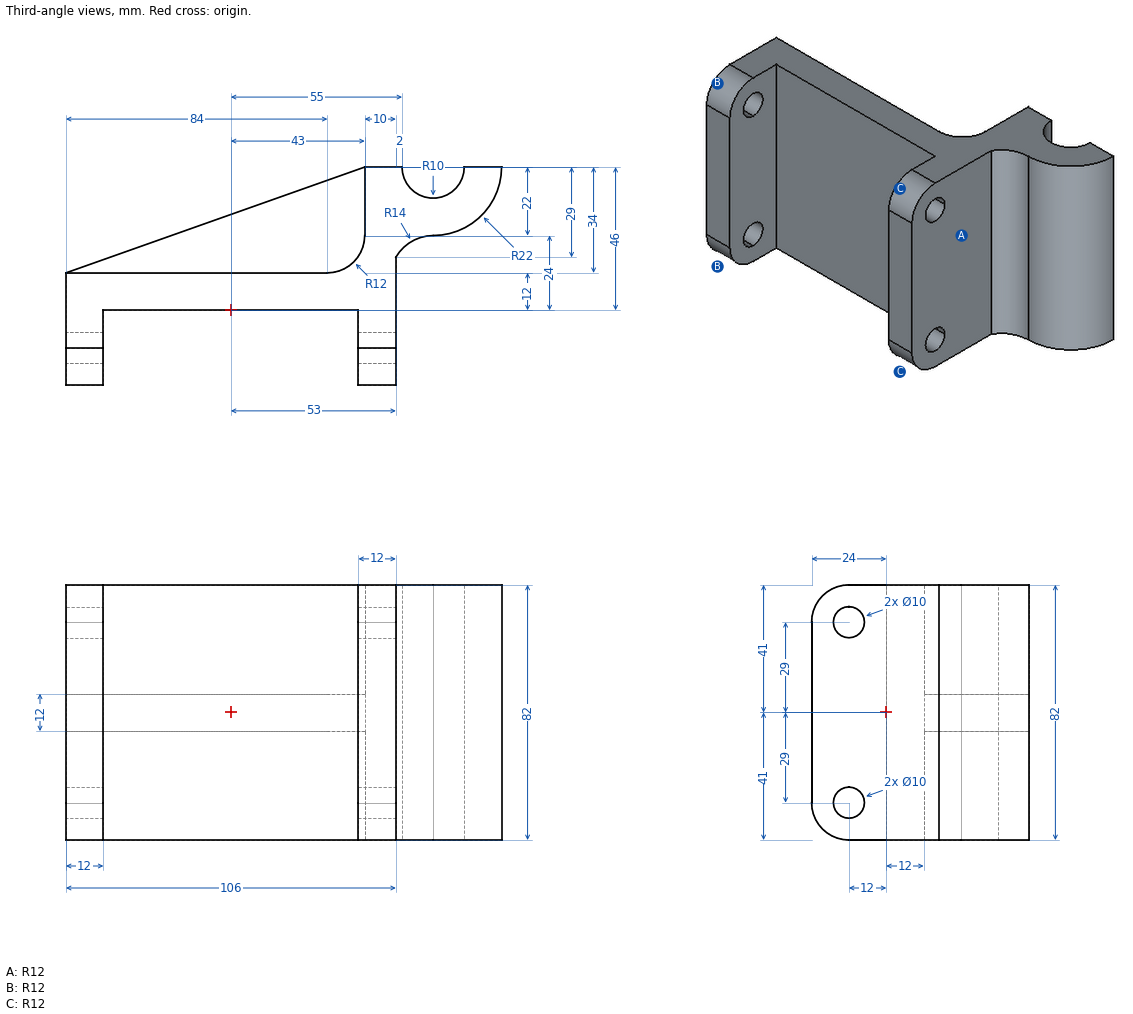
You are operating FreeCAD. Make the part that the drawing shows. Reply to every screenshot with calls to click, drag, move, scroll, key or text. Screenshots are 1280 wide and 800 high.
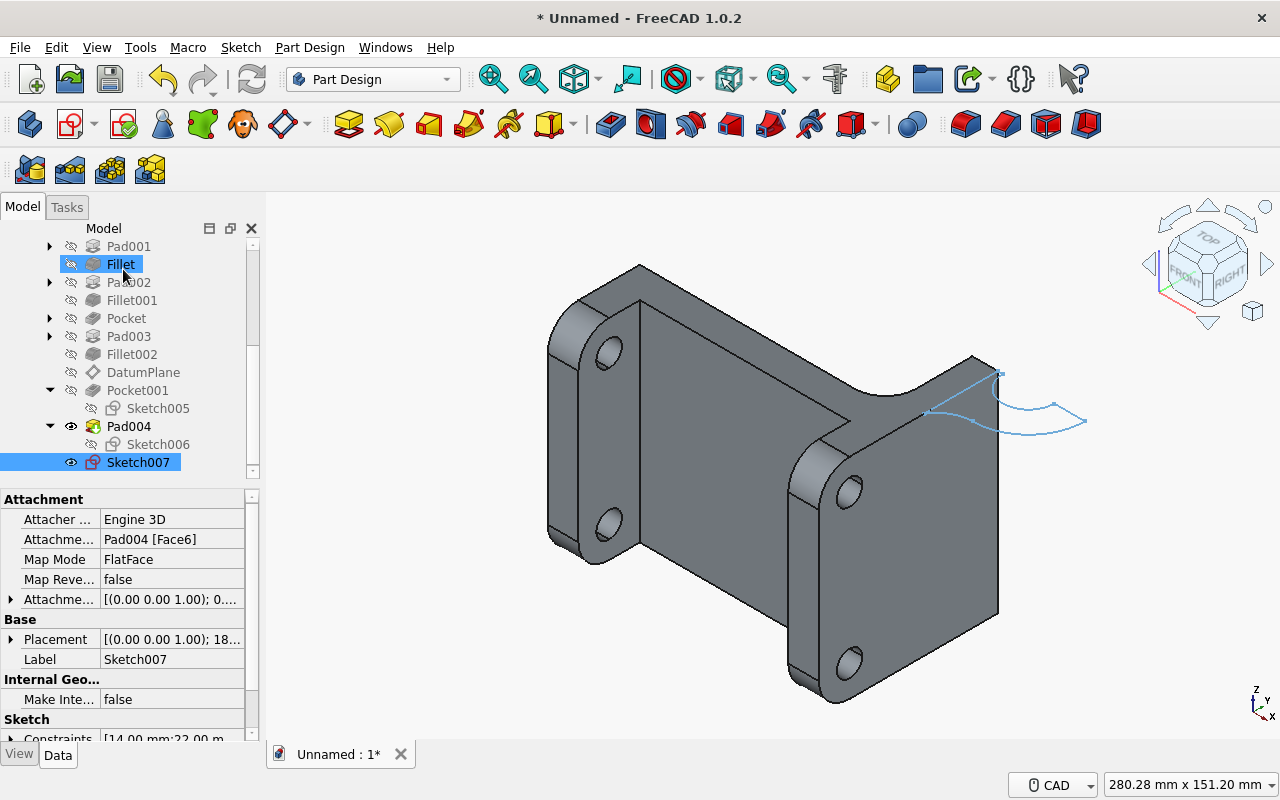
click(350, 124)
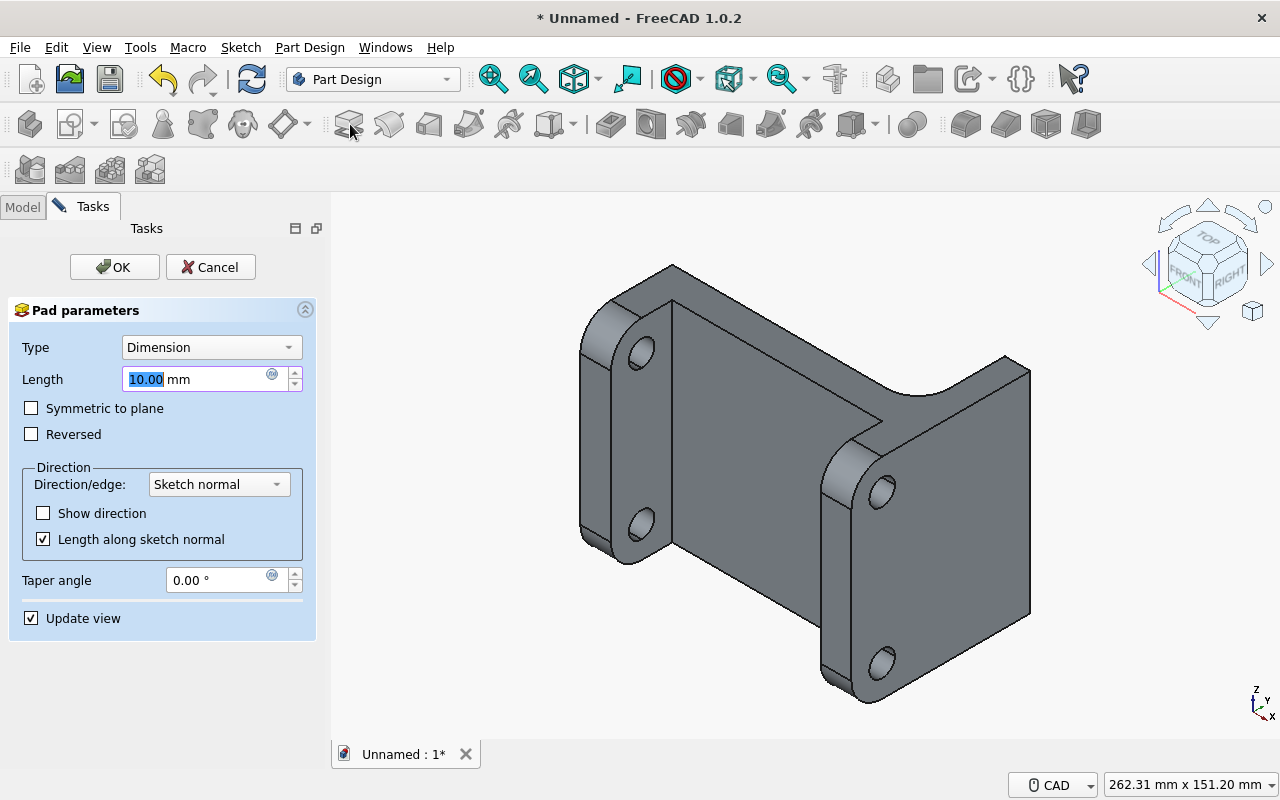
text(82)
key(Tab)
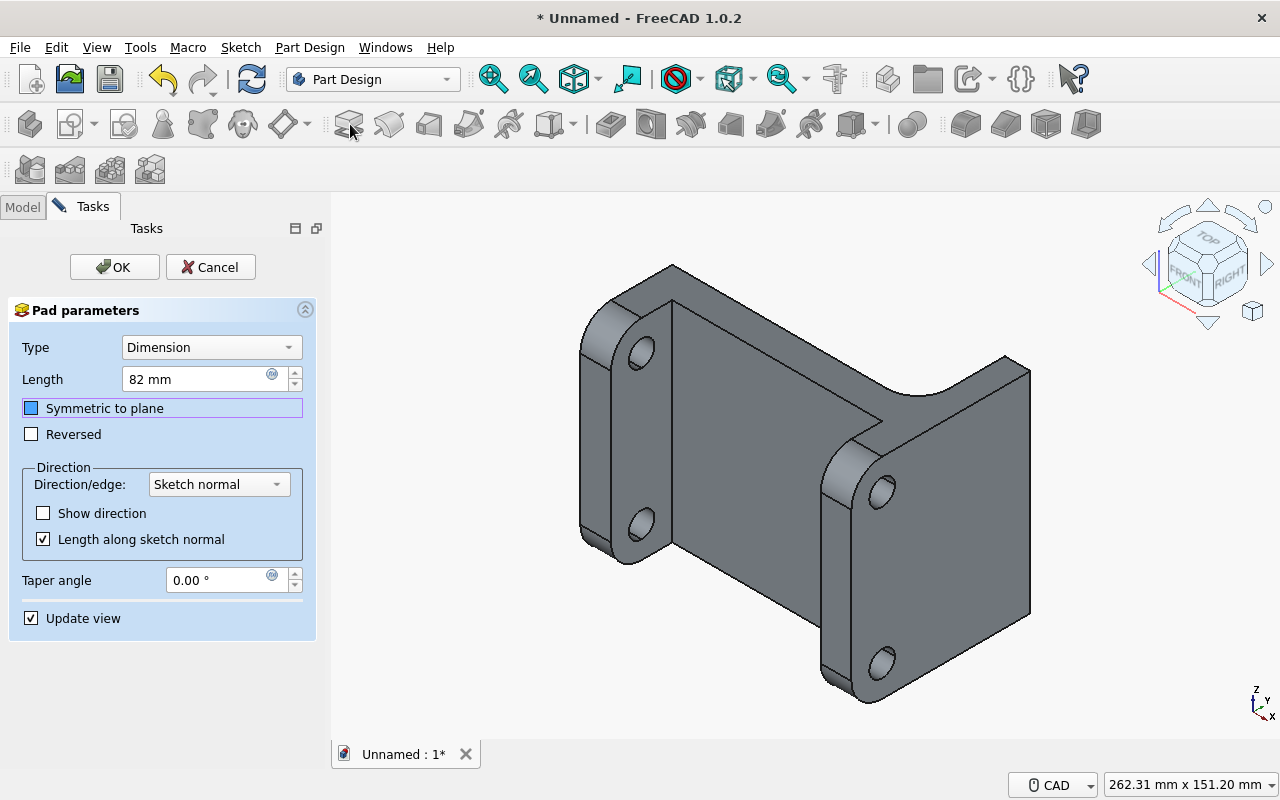
click(30, 434)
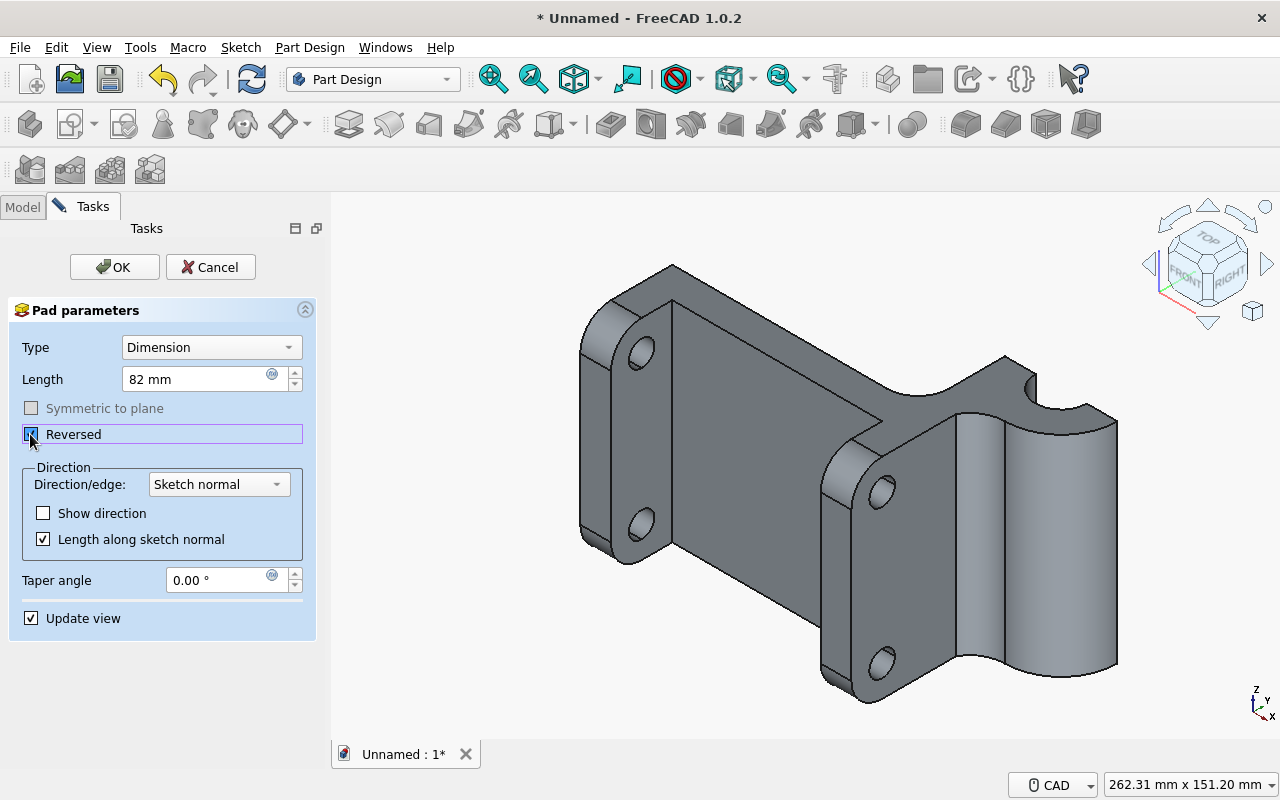
click(115, 267)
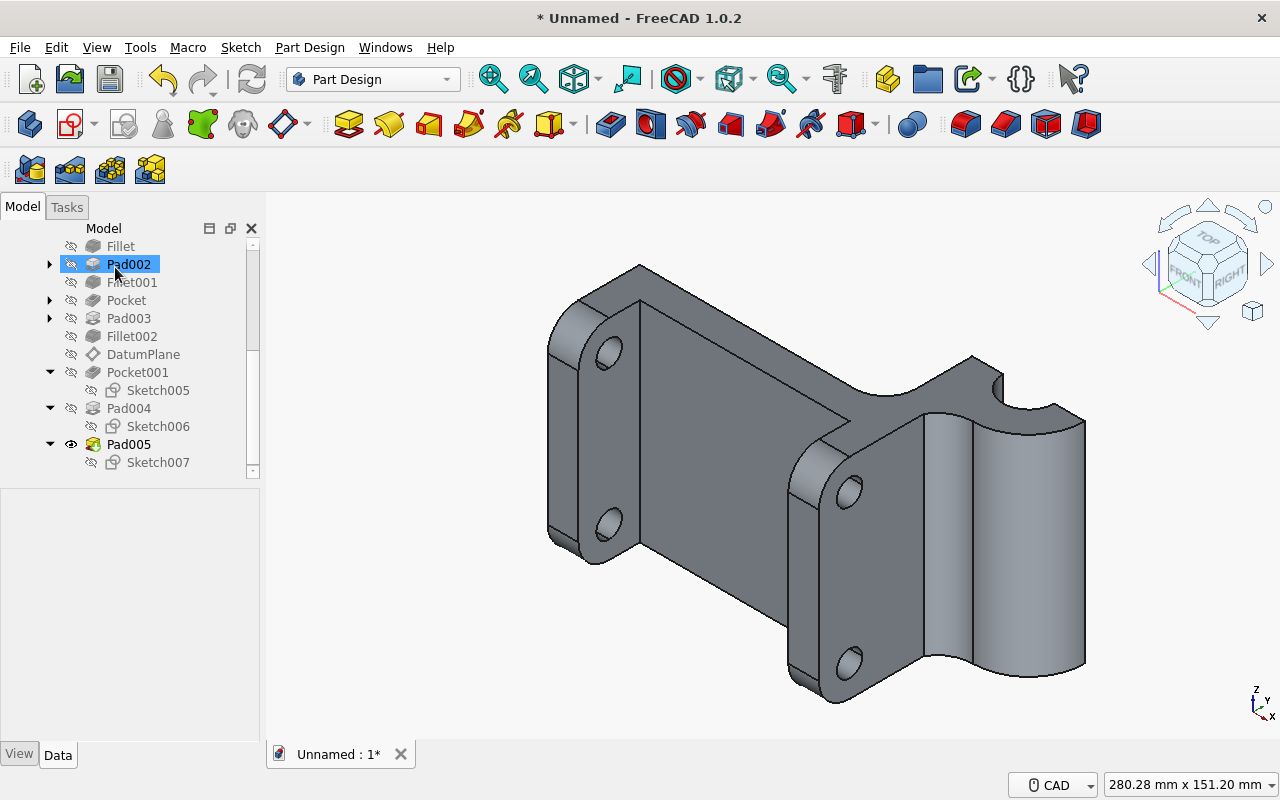
key(v)
key(f)